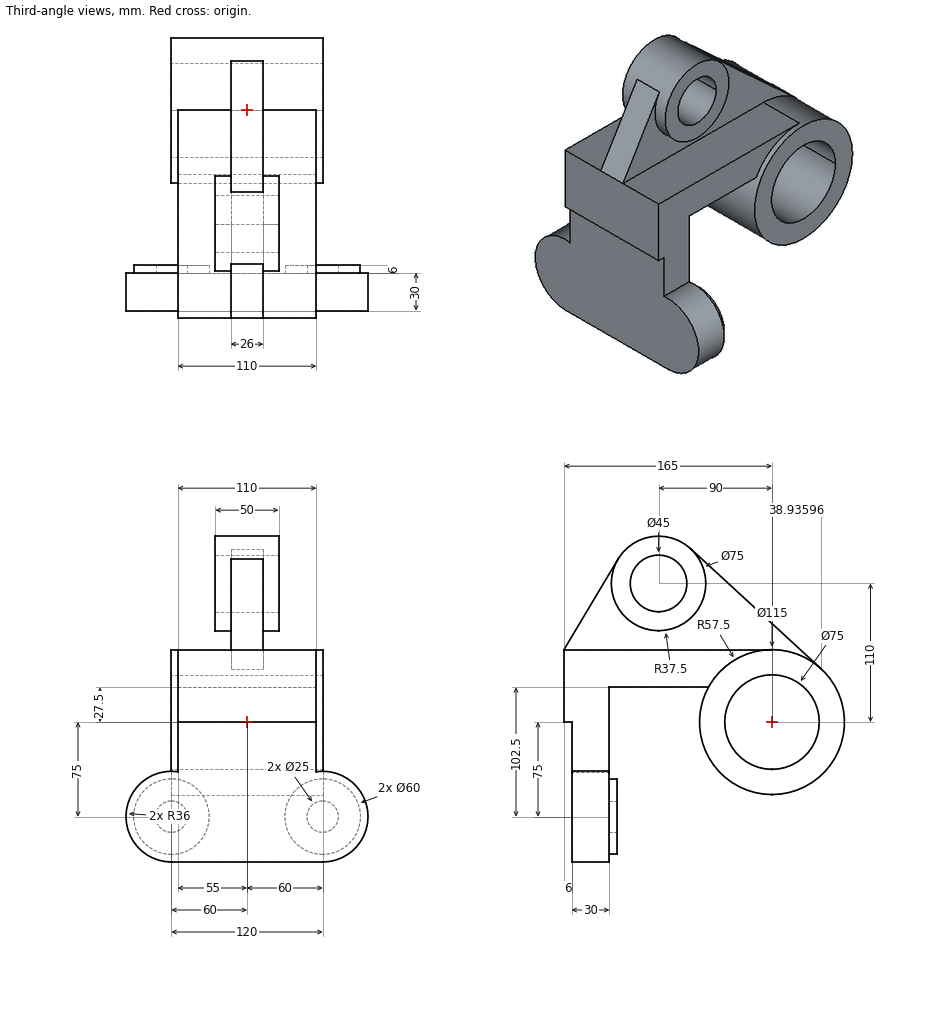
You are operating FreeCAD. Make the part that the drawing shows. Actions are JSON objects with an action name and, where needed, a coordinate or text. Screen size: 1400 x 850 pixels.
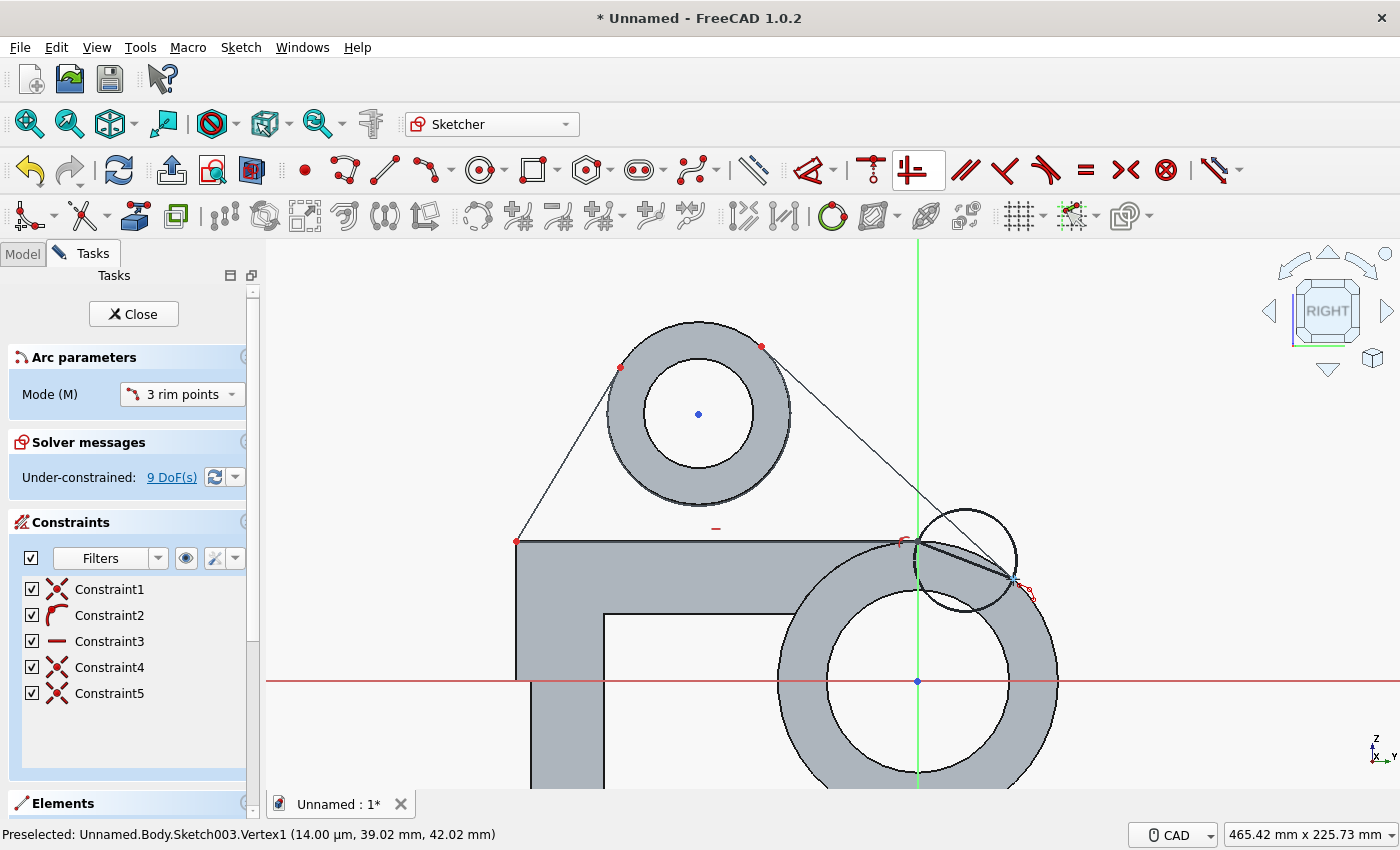
{"action": "scroll", "coordinate": [969, 551], "scroll_direction": "up", "scroll_amount": 3}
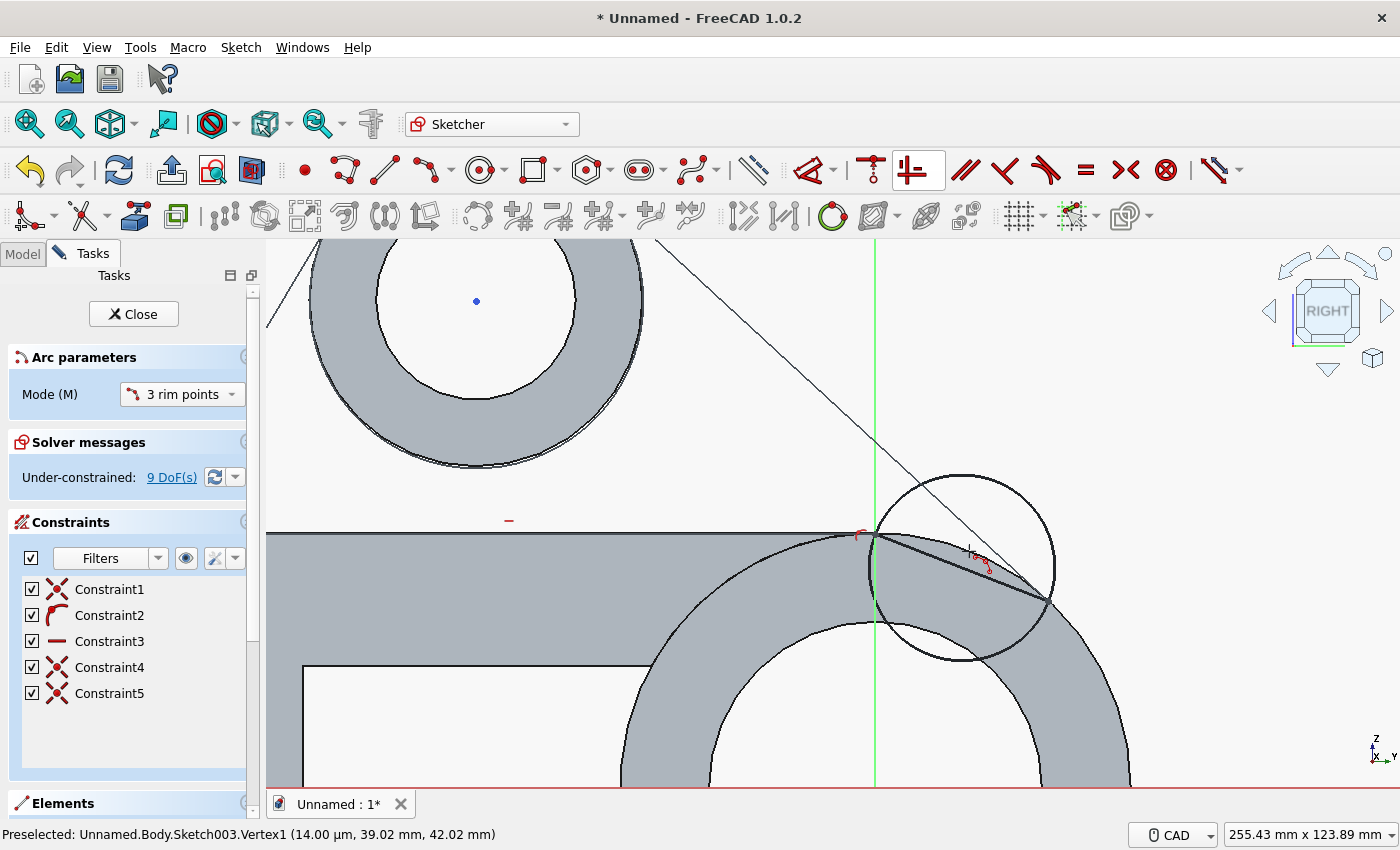
{"action": "left_click", "coordinate": [968, 550]}
{"action": "key", "text": "Escape"}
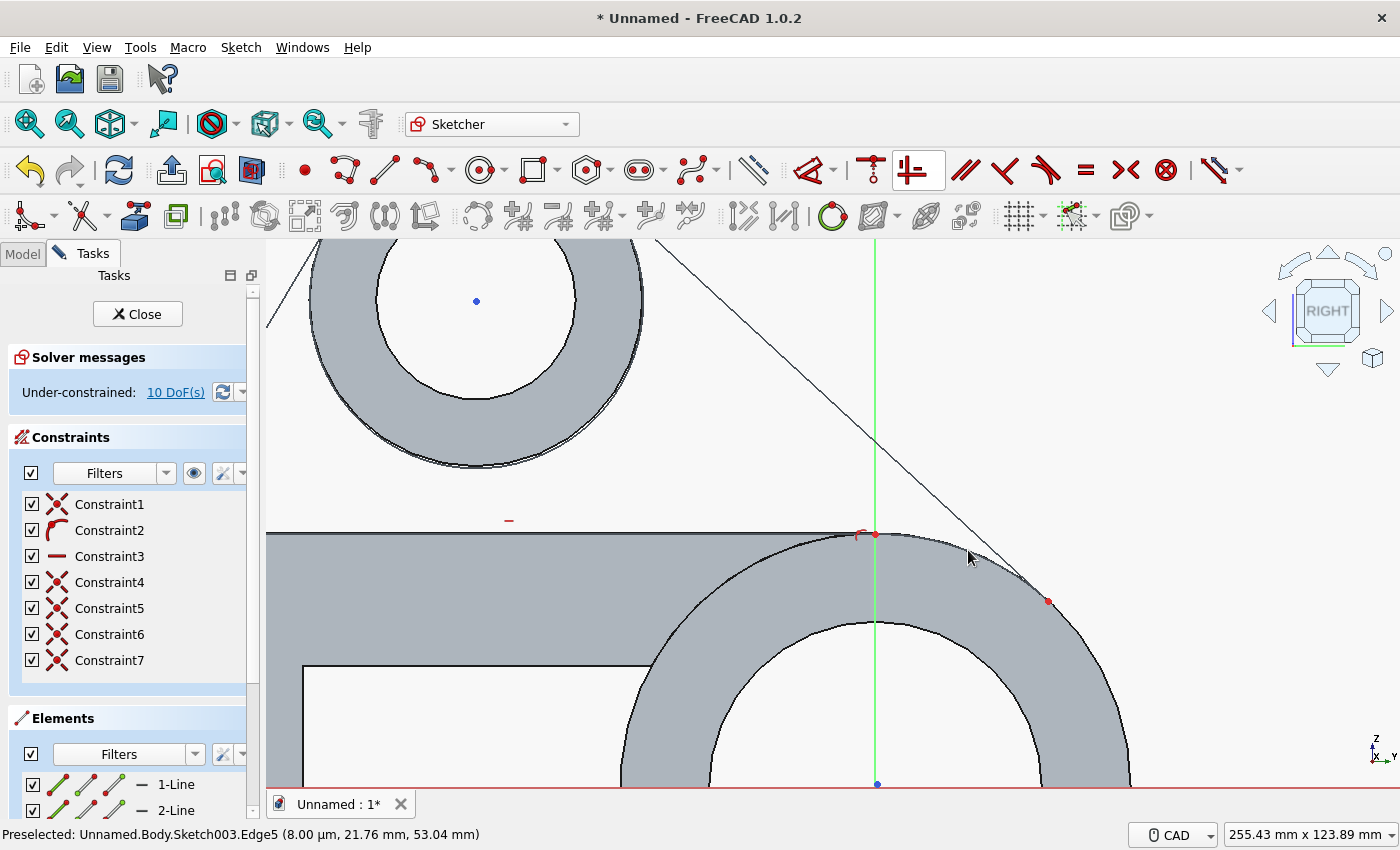
{"action": "left_click", "coordinate": [911, 475]}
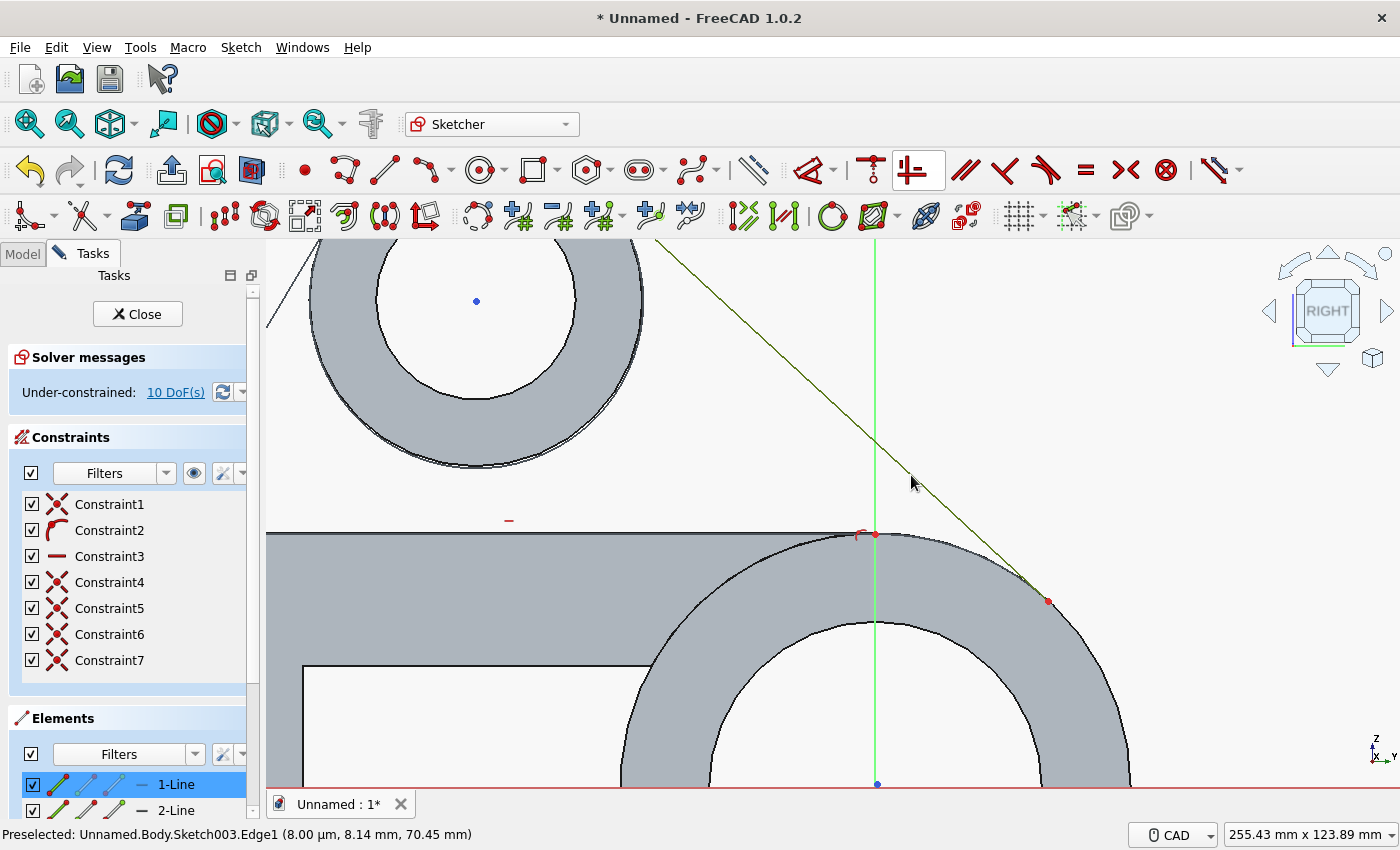
{"action": "left_click", "coordinate": [362, 423]}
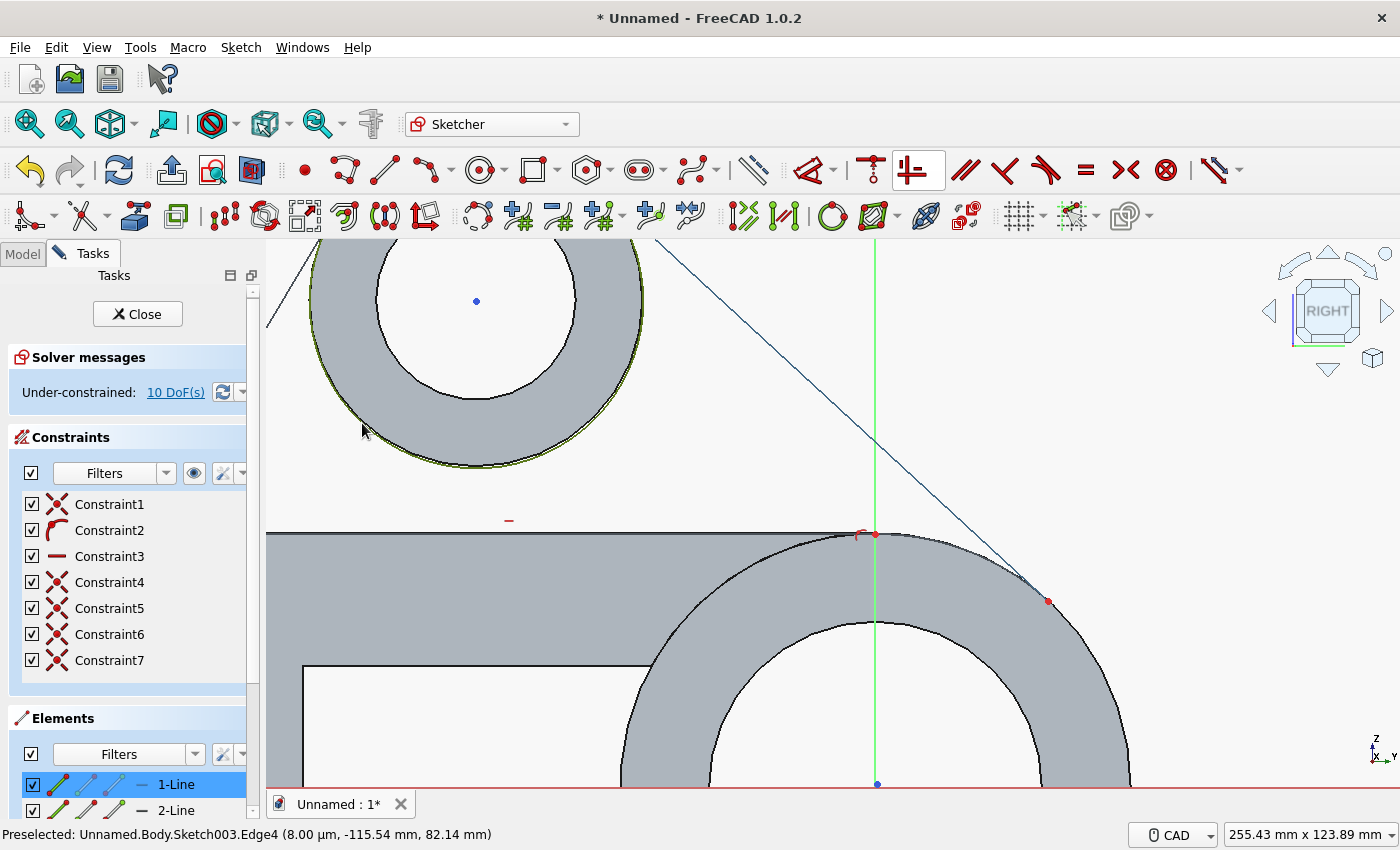
{"action": "left_click", "coordinate": [1046, 170]}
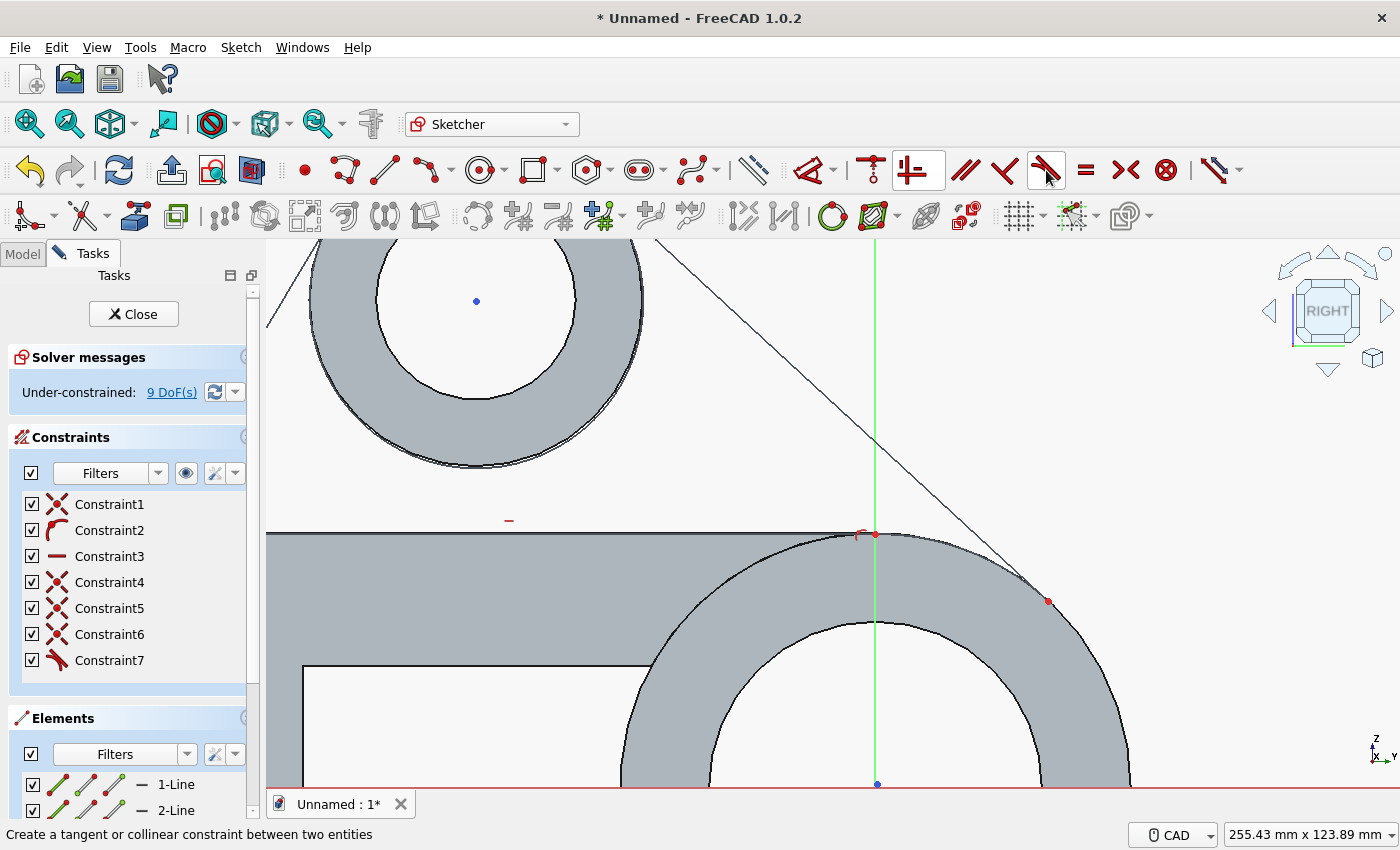
{"action": "left_click", "coordinate": [295, 280]}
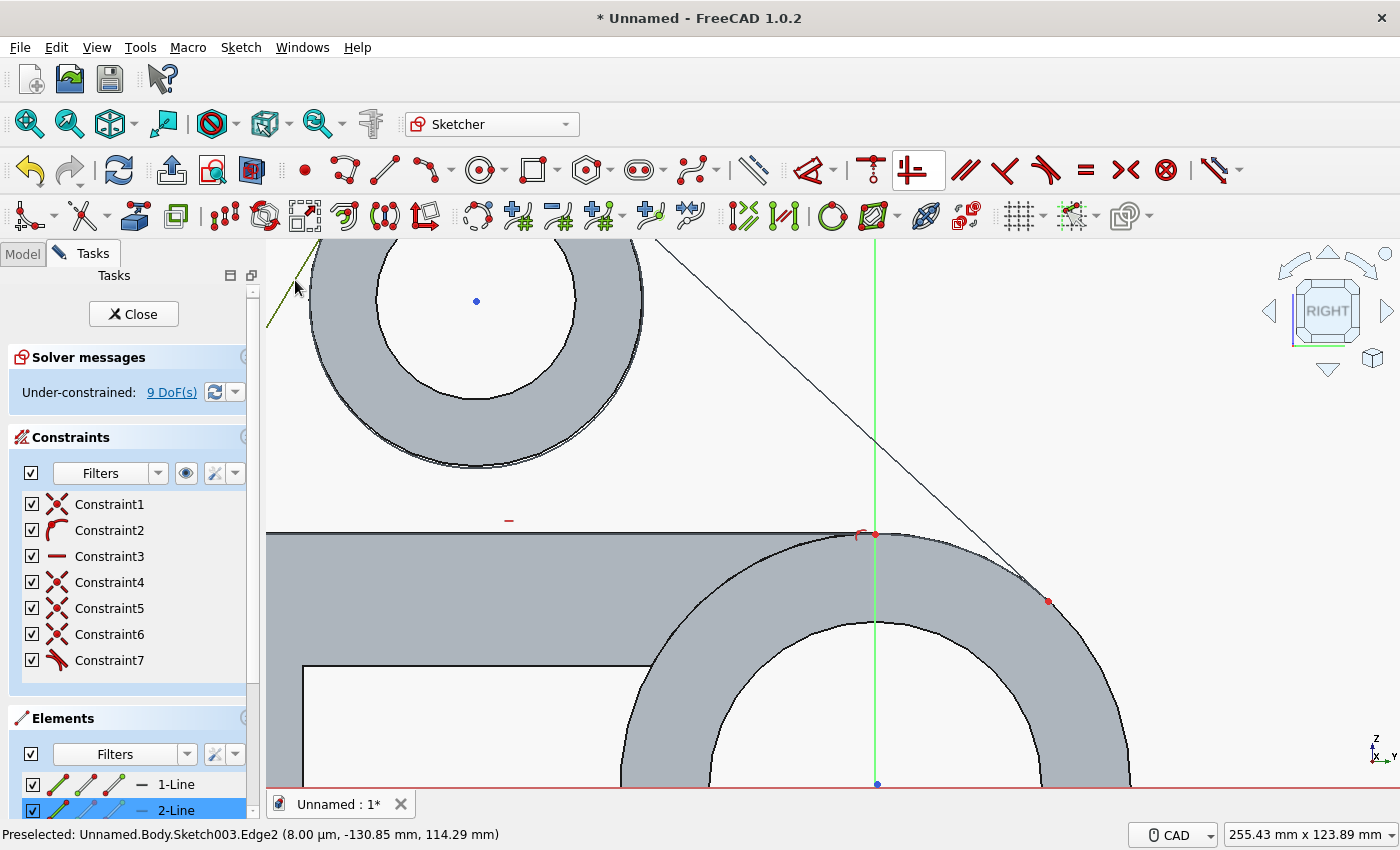
{"action": "left_click", "coordinate": [362, 423]}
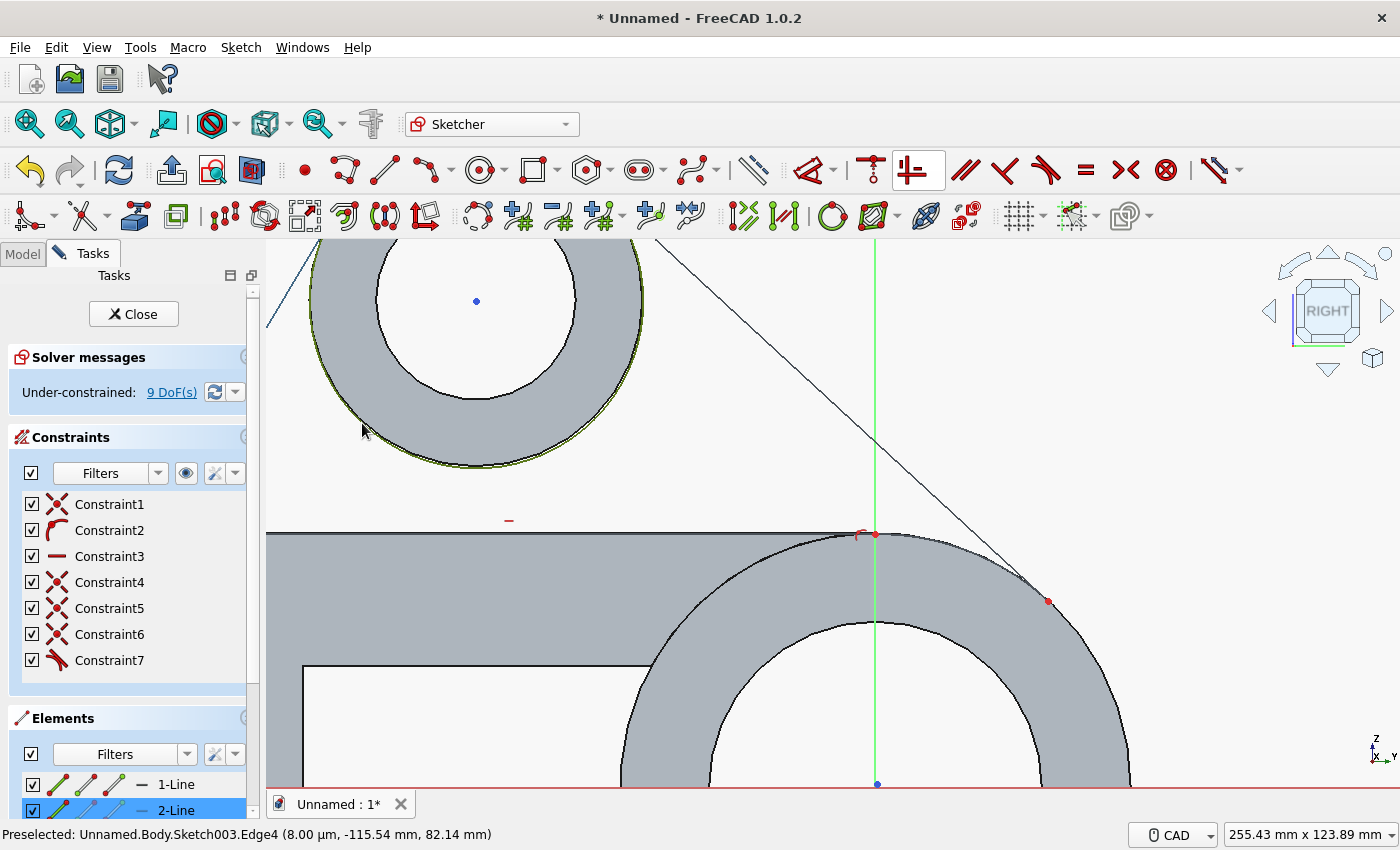
{"action": "key", "text": "t"}